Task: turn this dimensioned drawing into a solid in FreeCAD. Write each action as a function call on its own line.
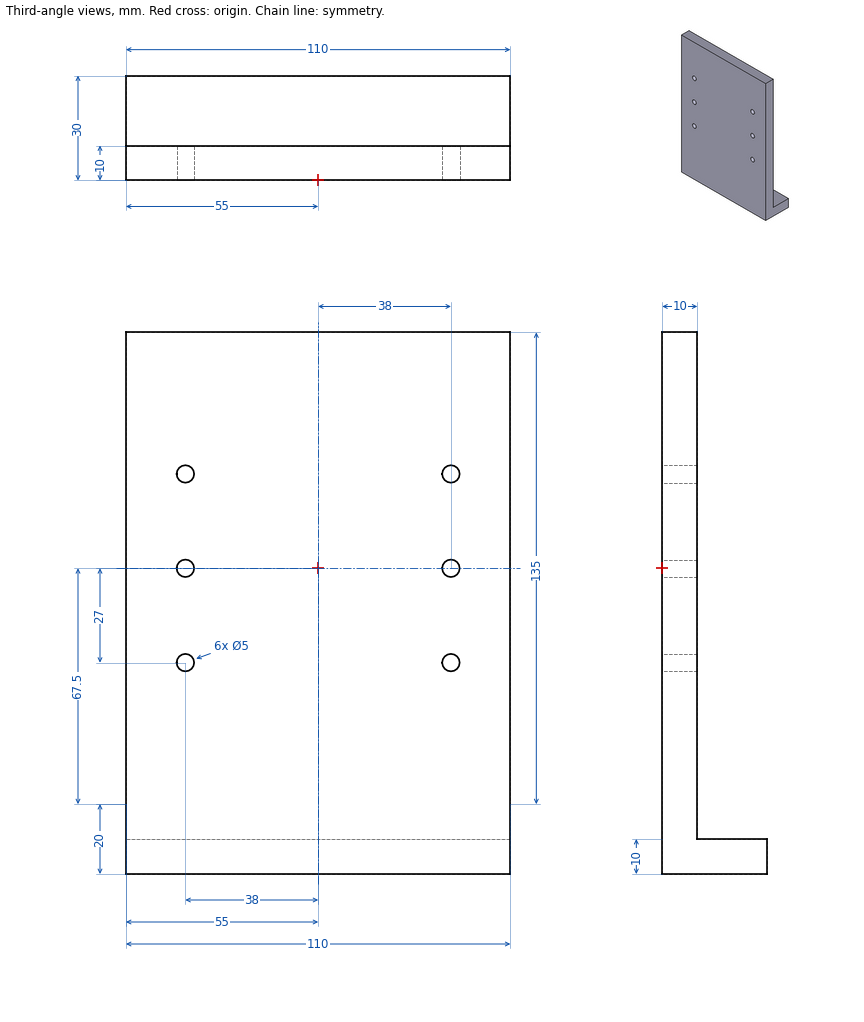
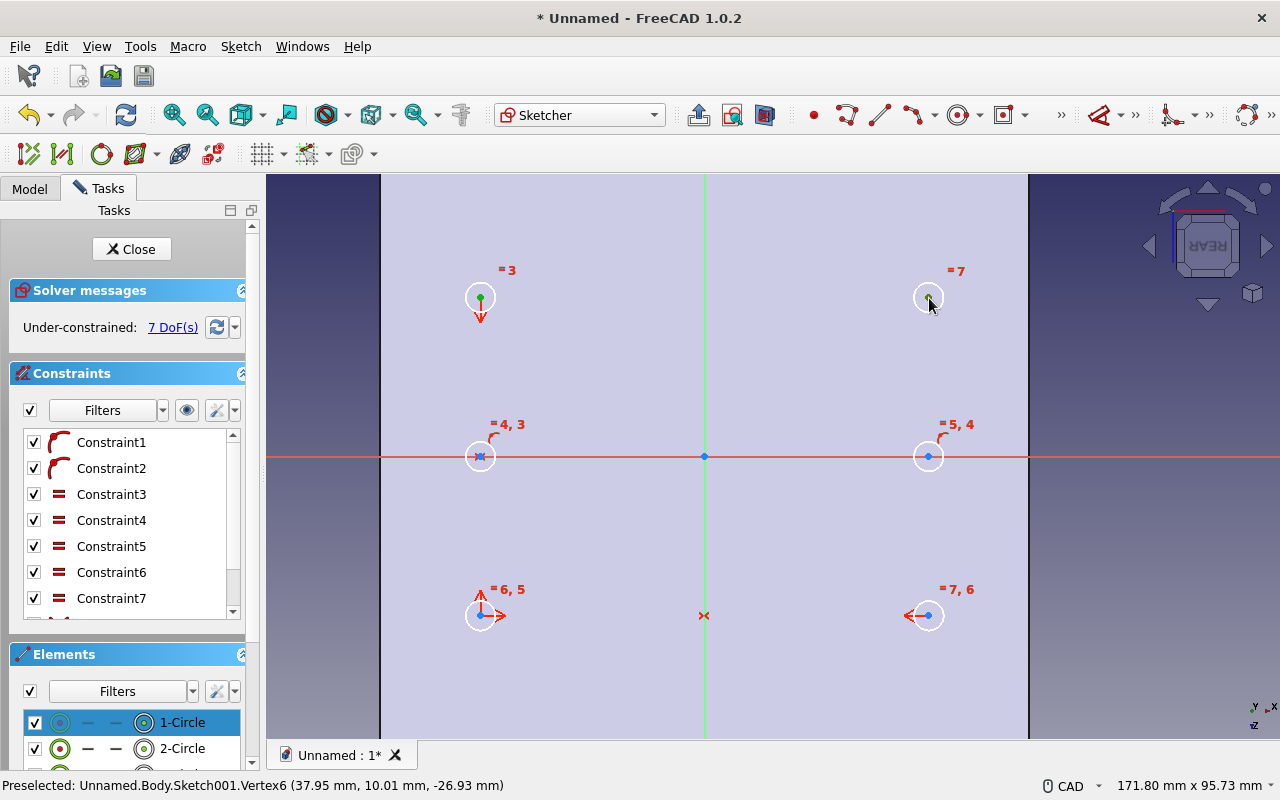
click(705, 675)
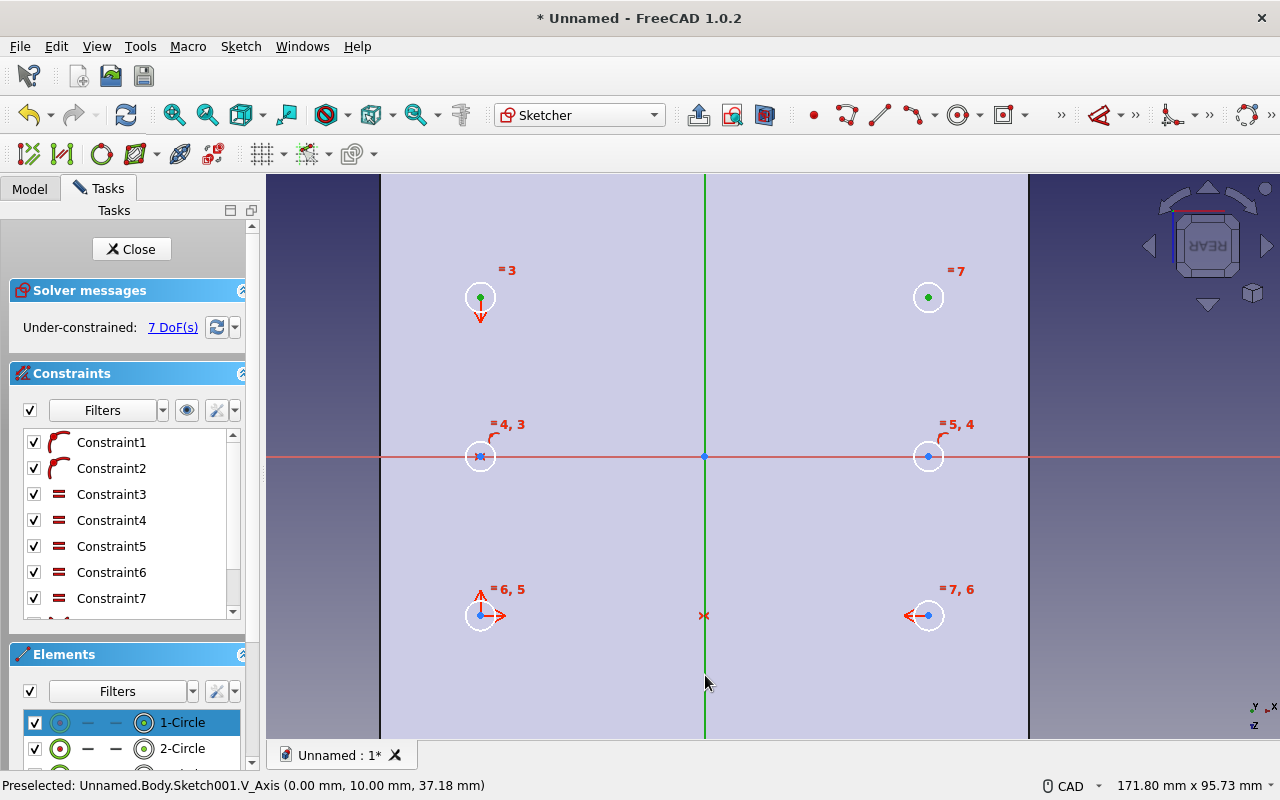
key(s)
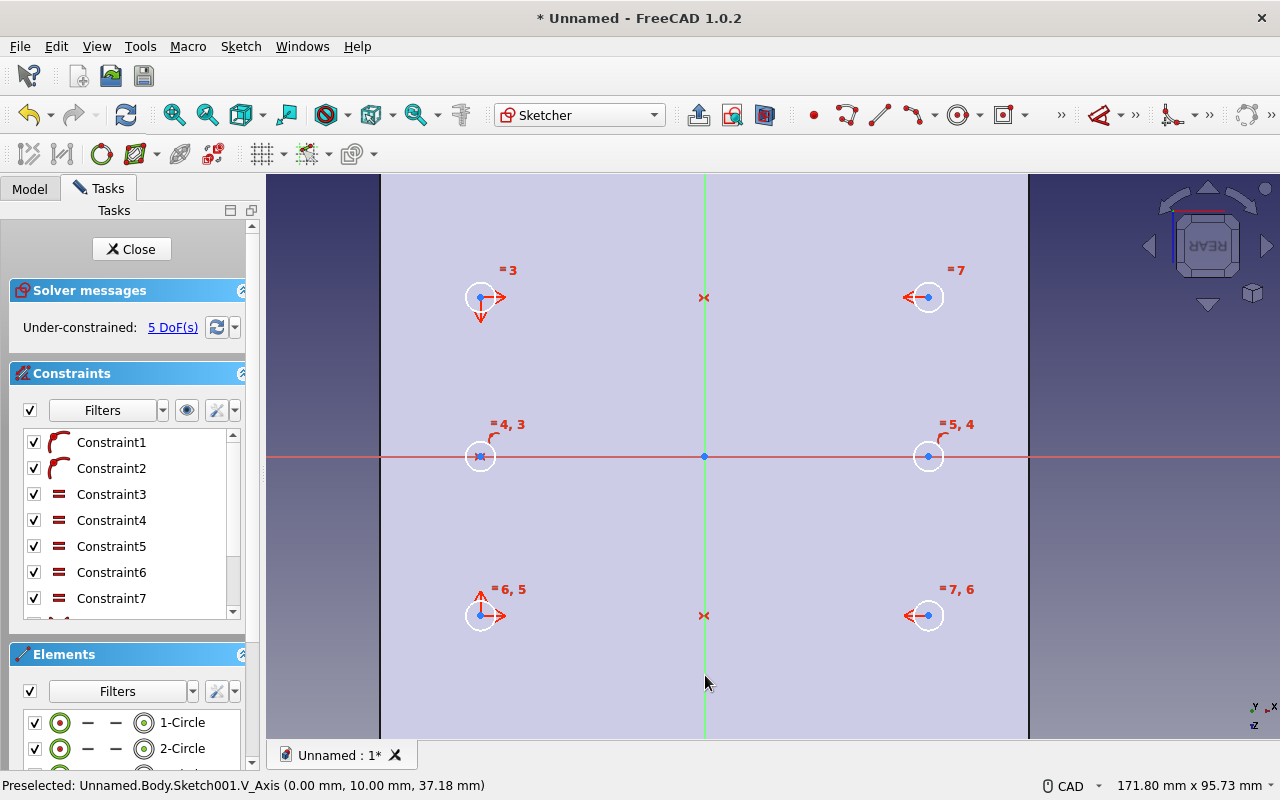
click(1098, 116)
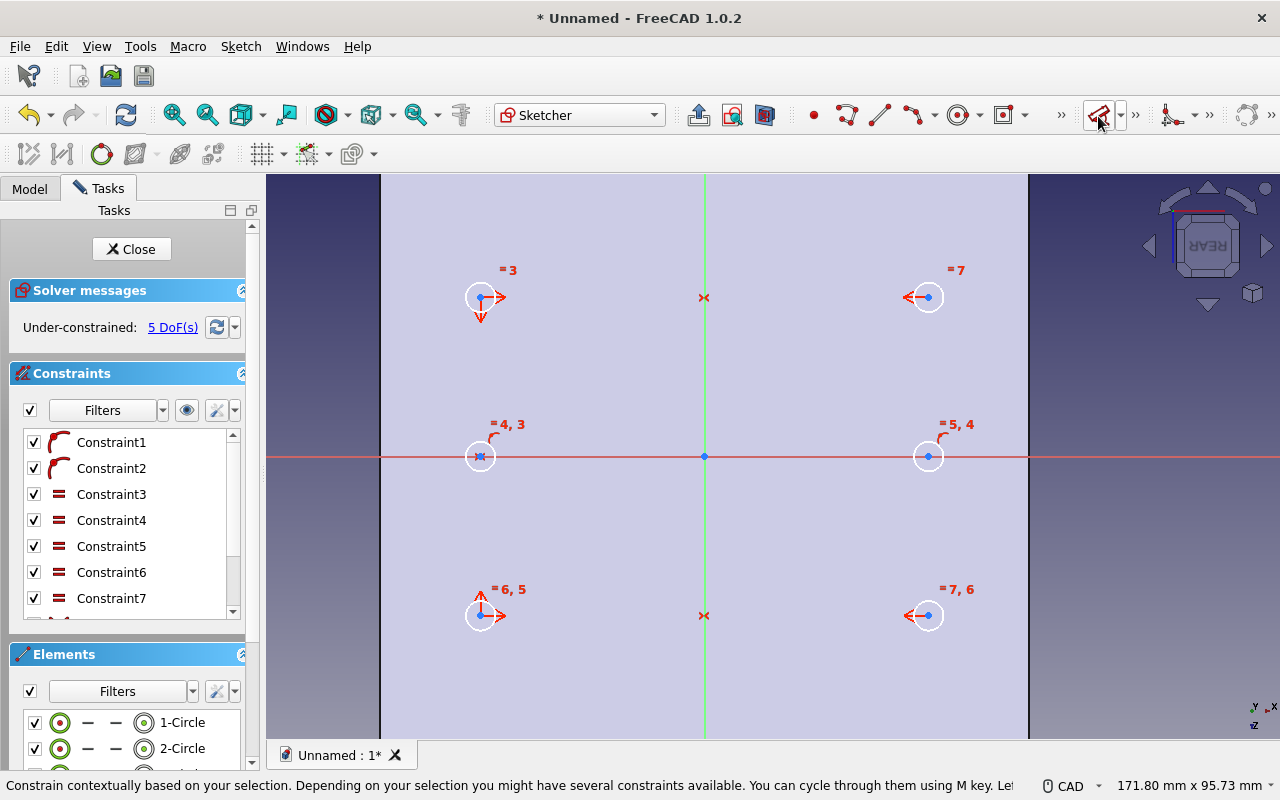
scroll(491, 287, up, 2)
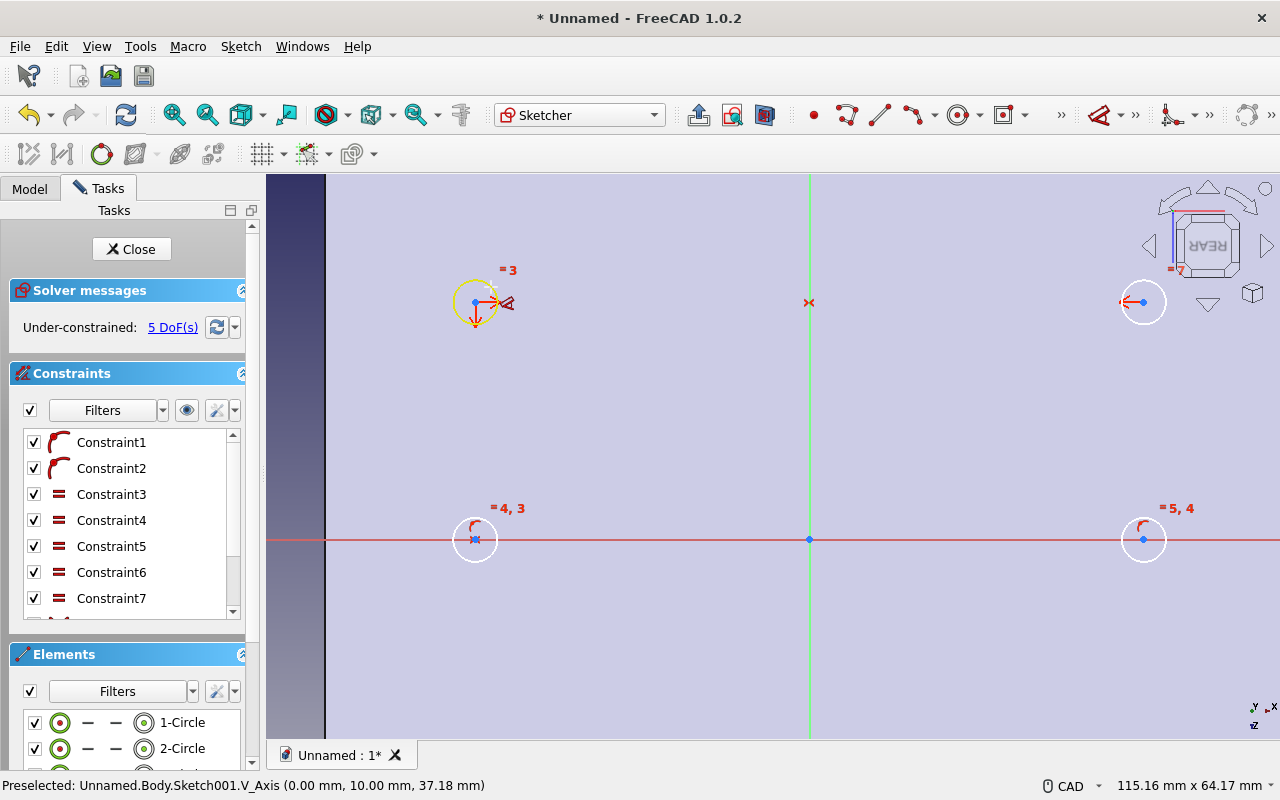
click(491, 287)
click(514, 264)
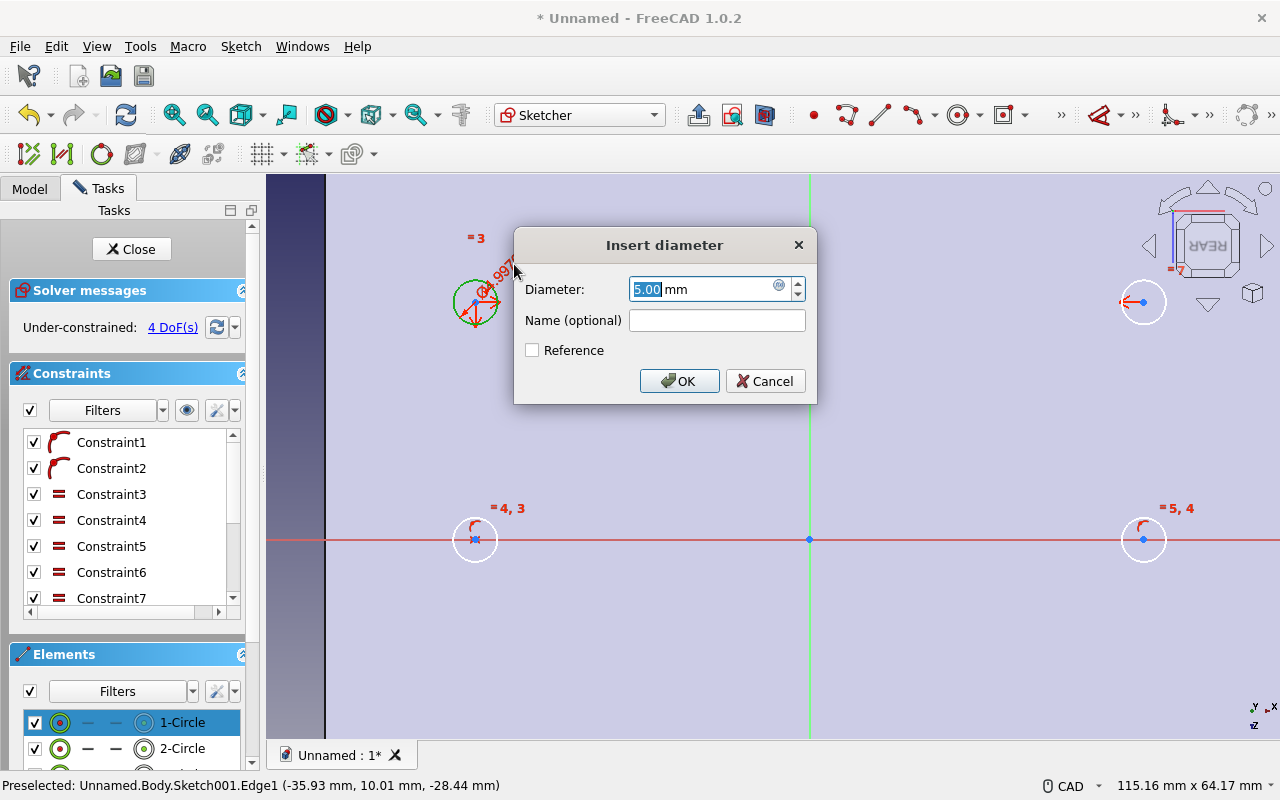
text(5)
key(Return)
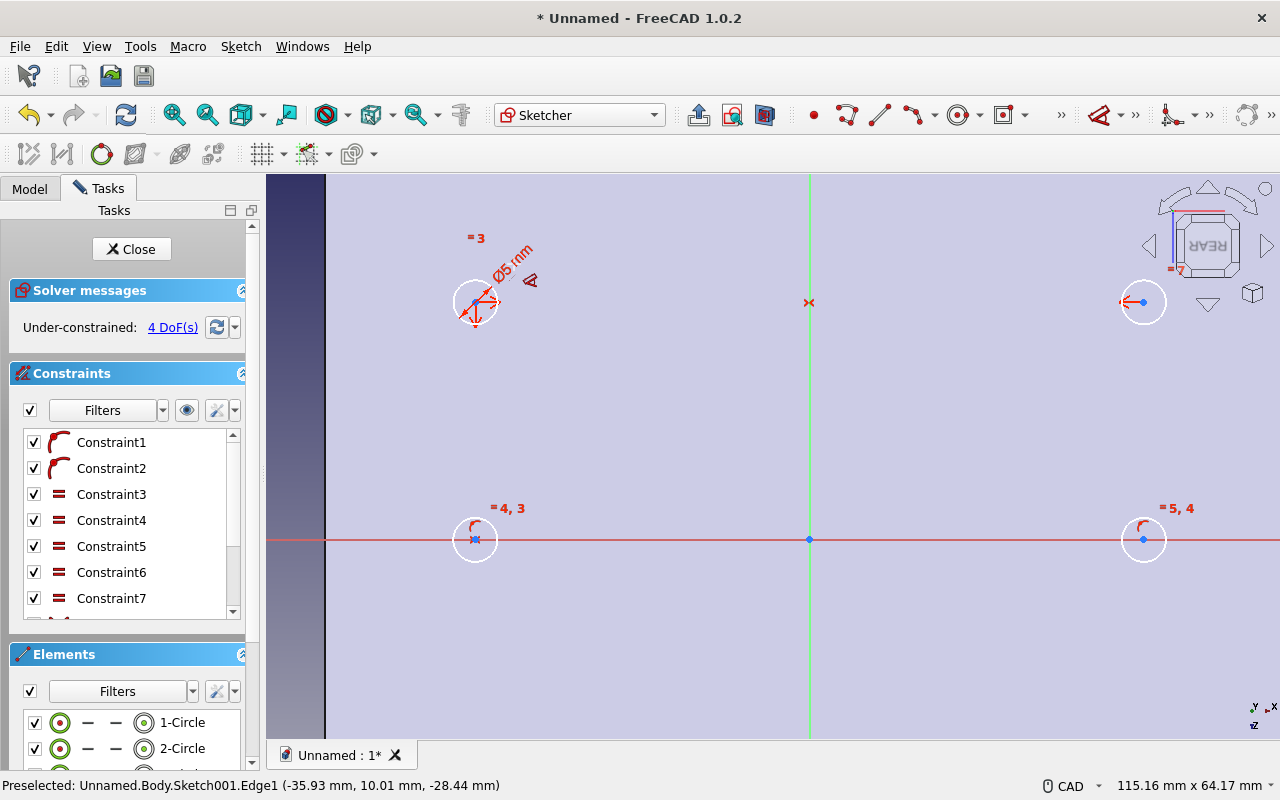
click(476, 302)
click(643, 268)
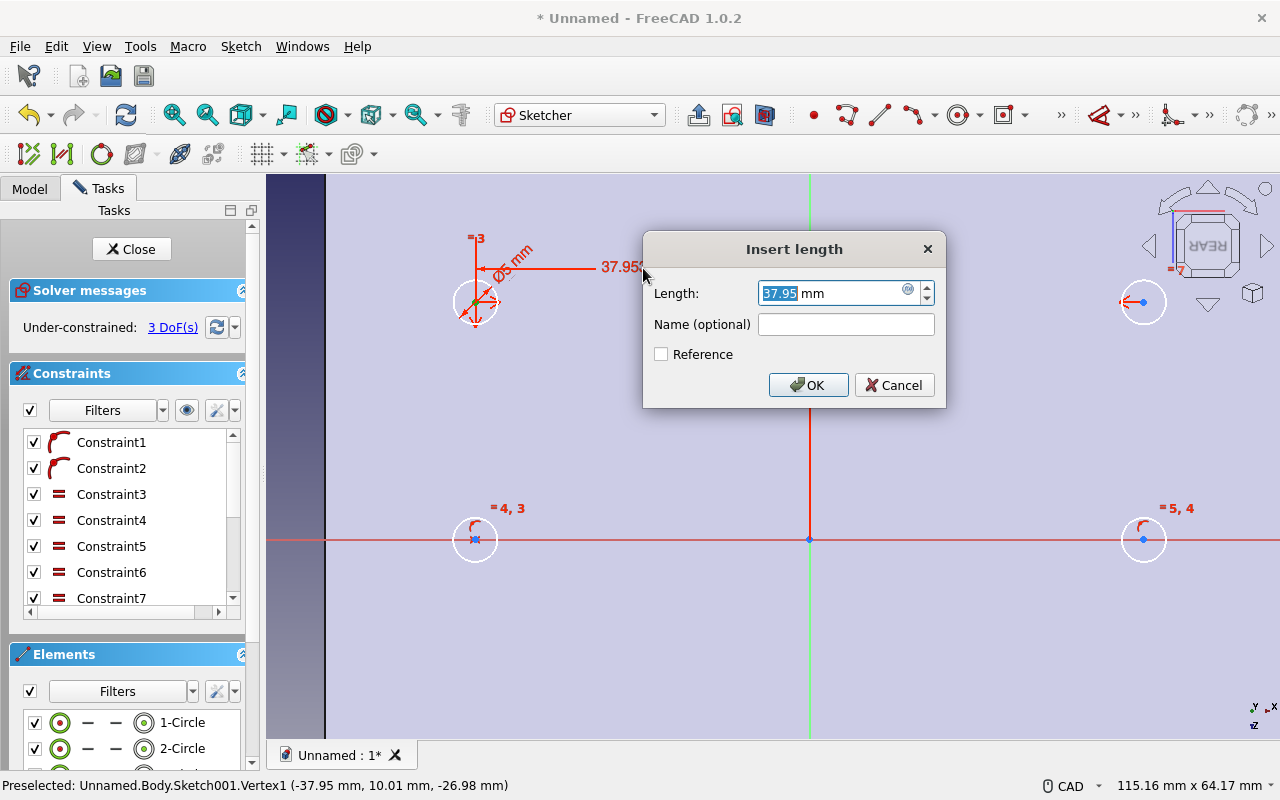
text(38)
key(Return)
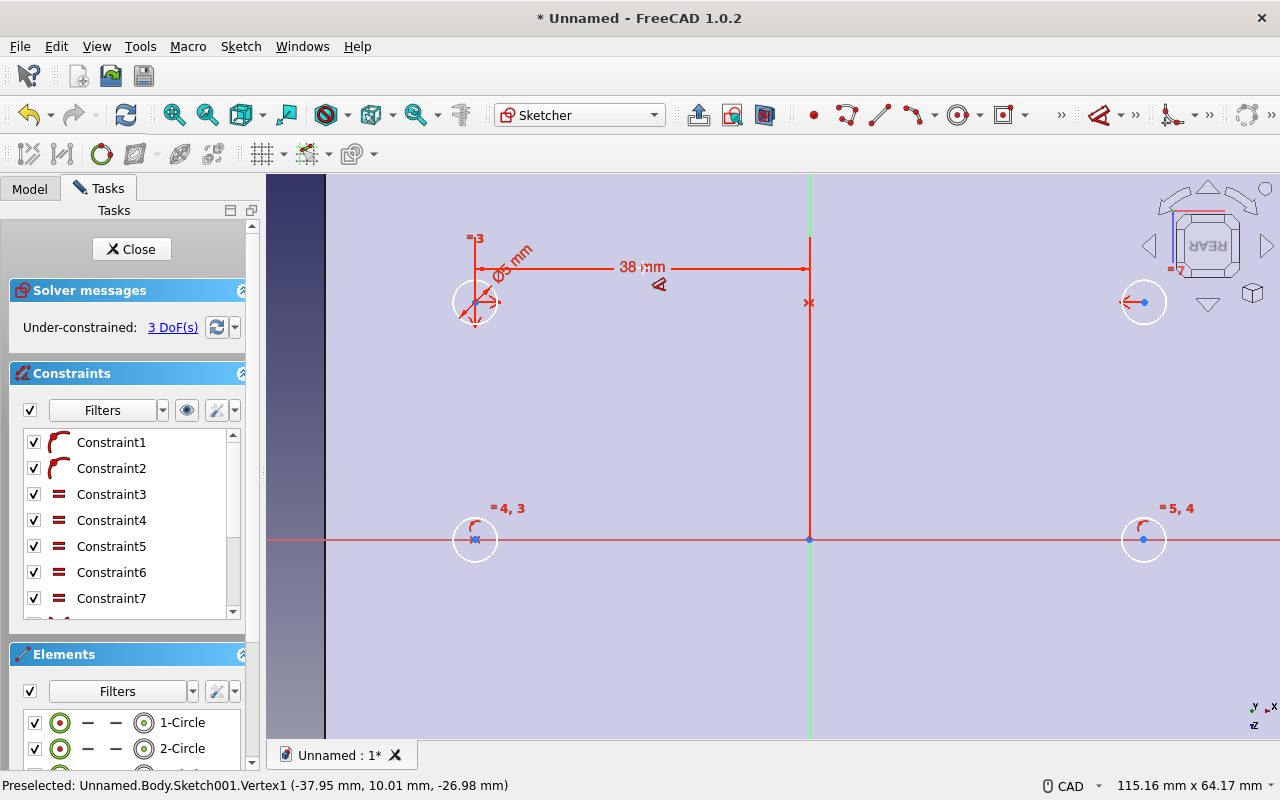
click(475, 302)
click(441, 421)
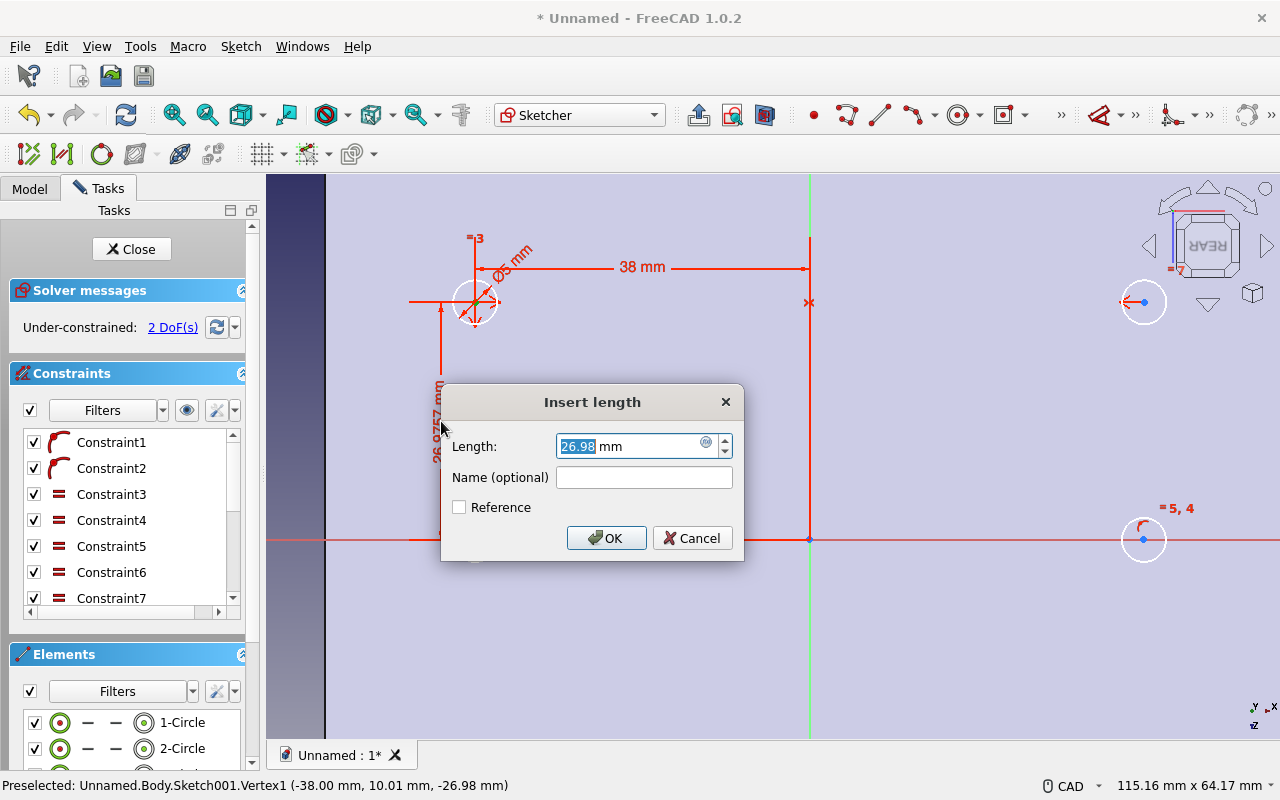
text(27)
key(Return)